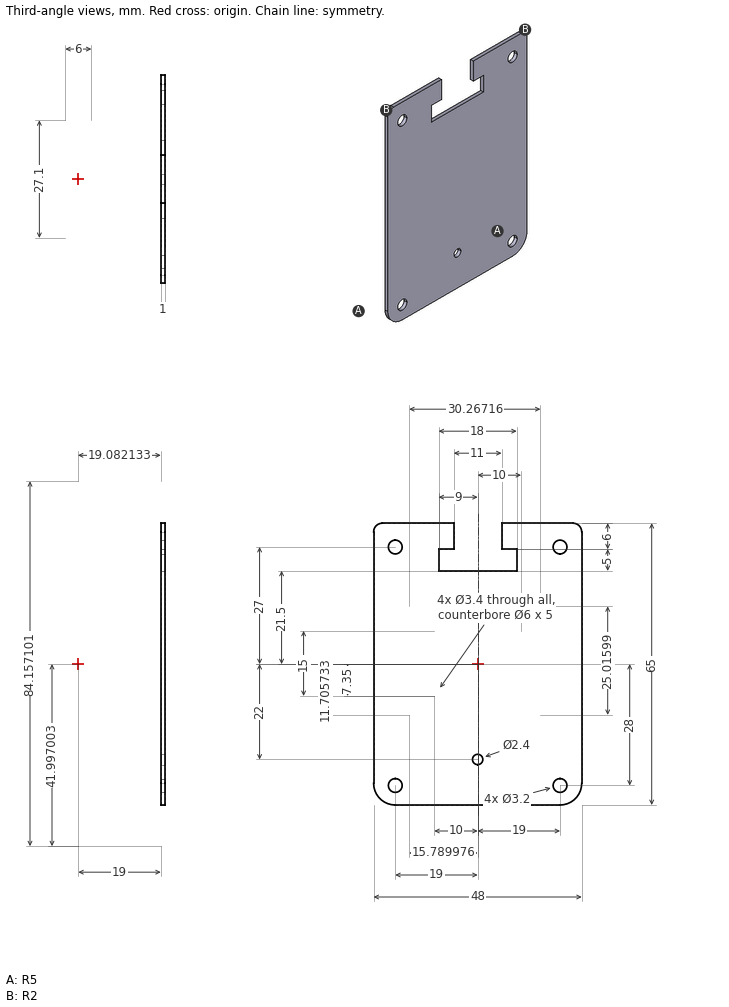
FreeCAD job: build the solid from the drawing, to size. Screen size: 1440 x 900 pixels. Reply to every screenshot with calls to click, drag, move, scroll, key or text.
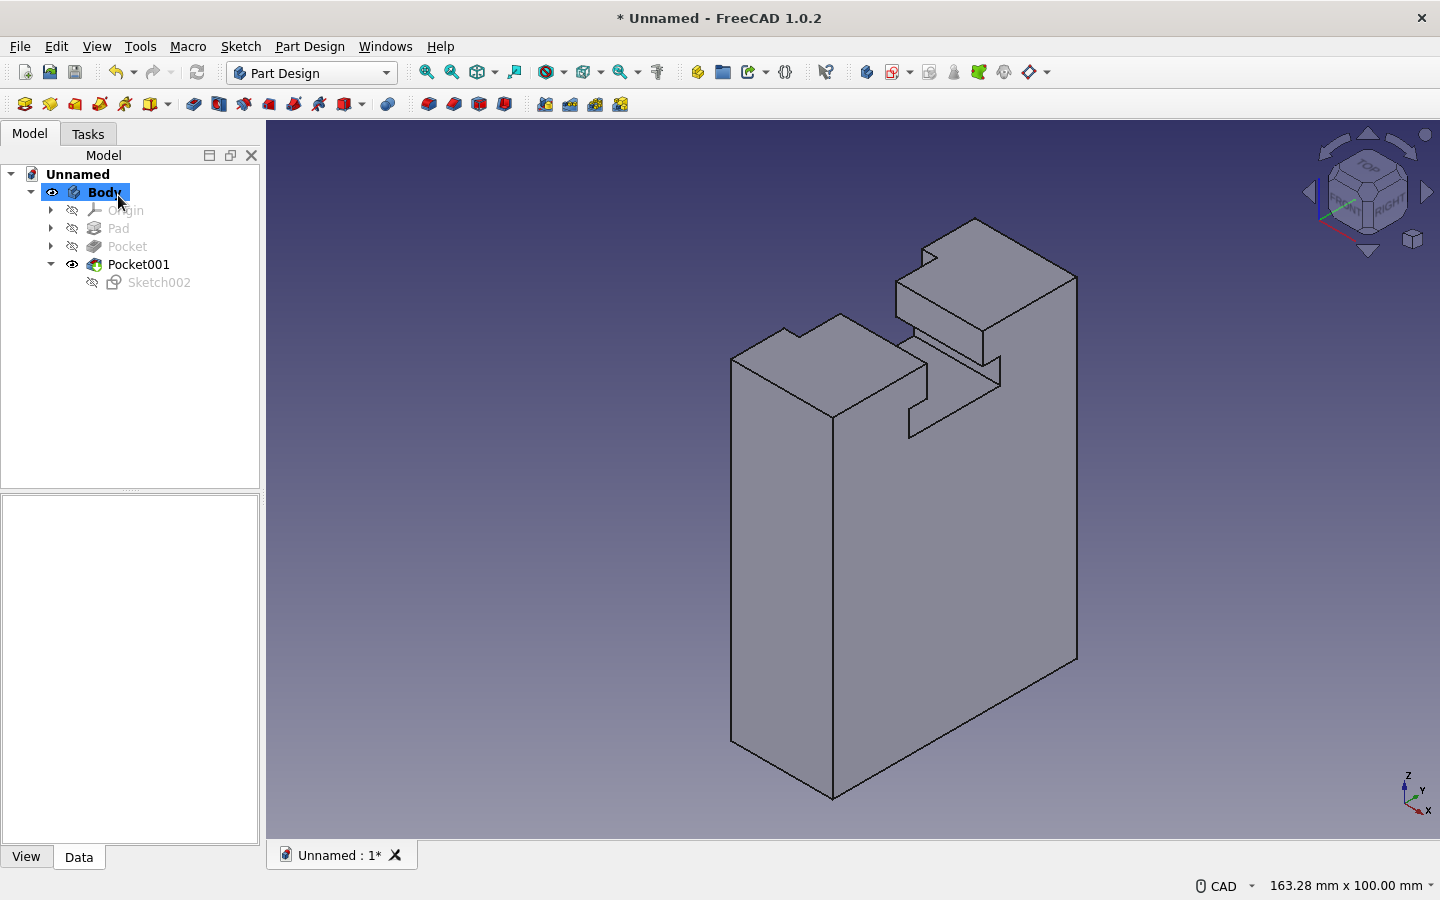
click(955, 592)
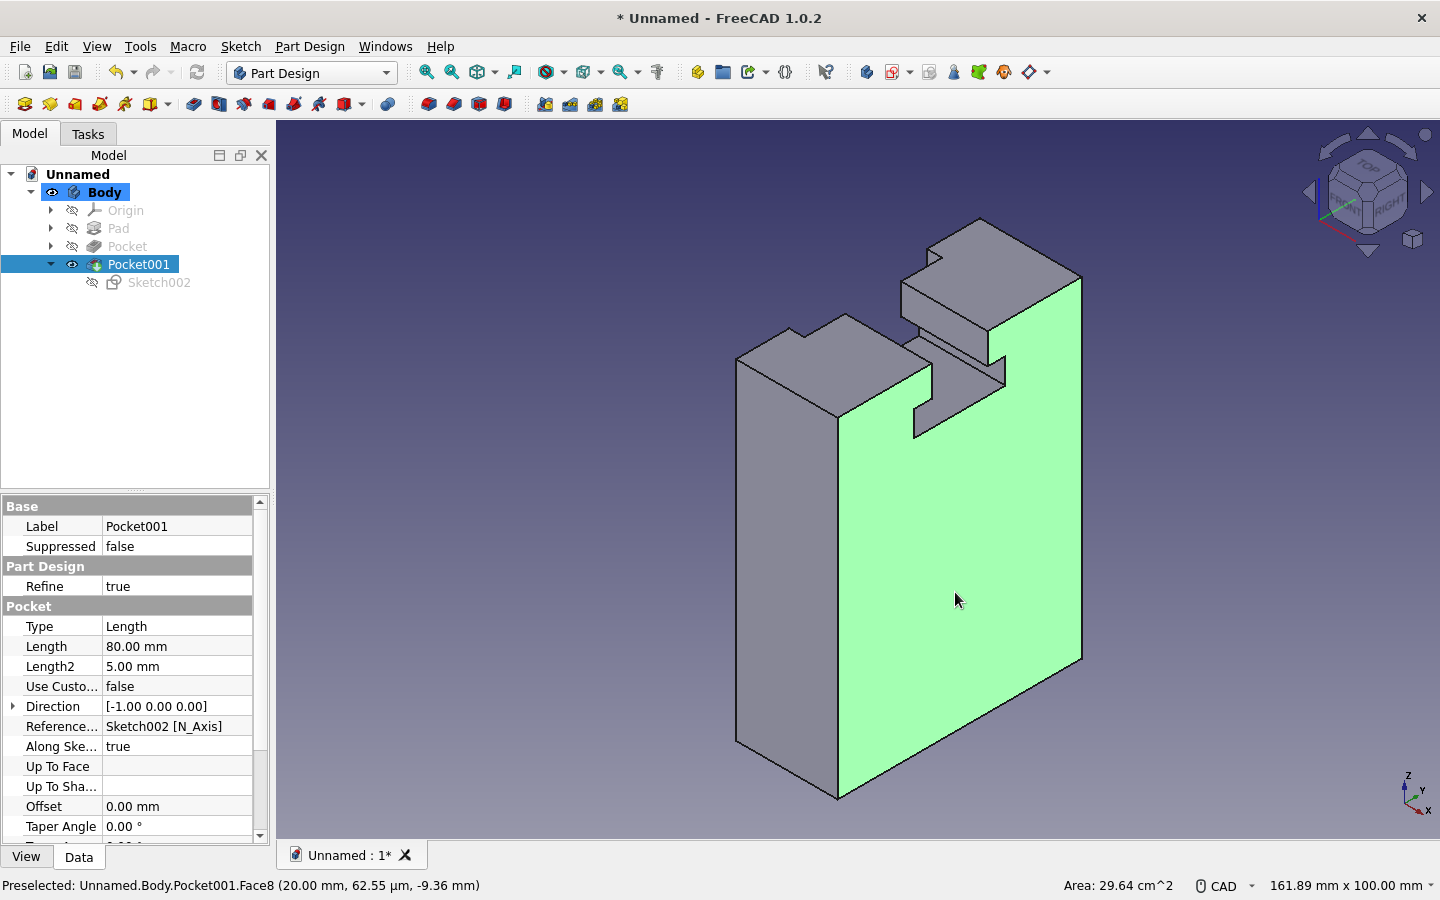
click(892, 72)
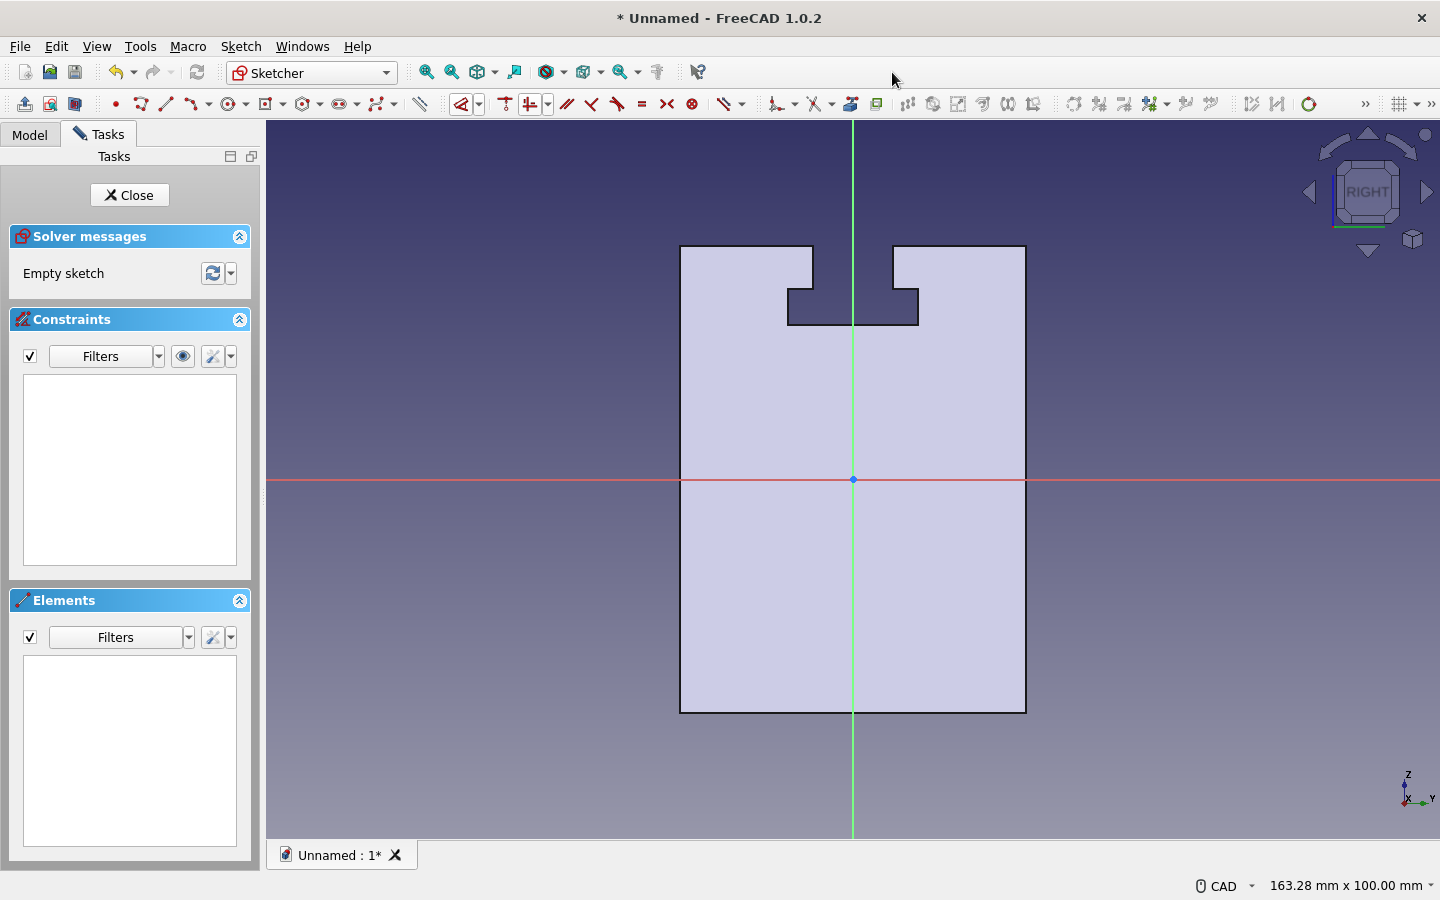
scroll(857, 646, up, 15)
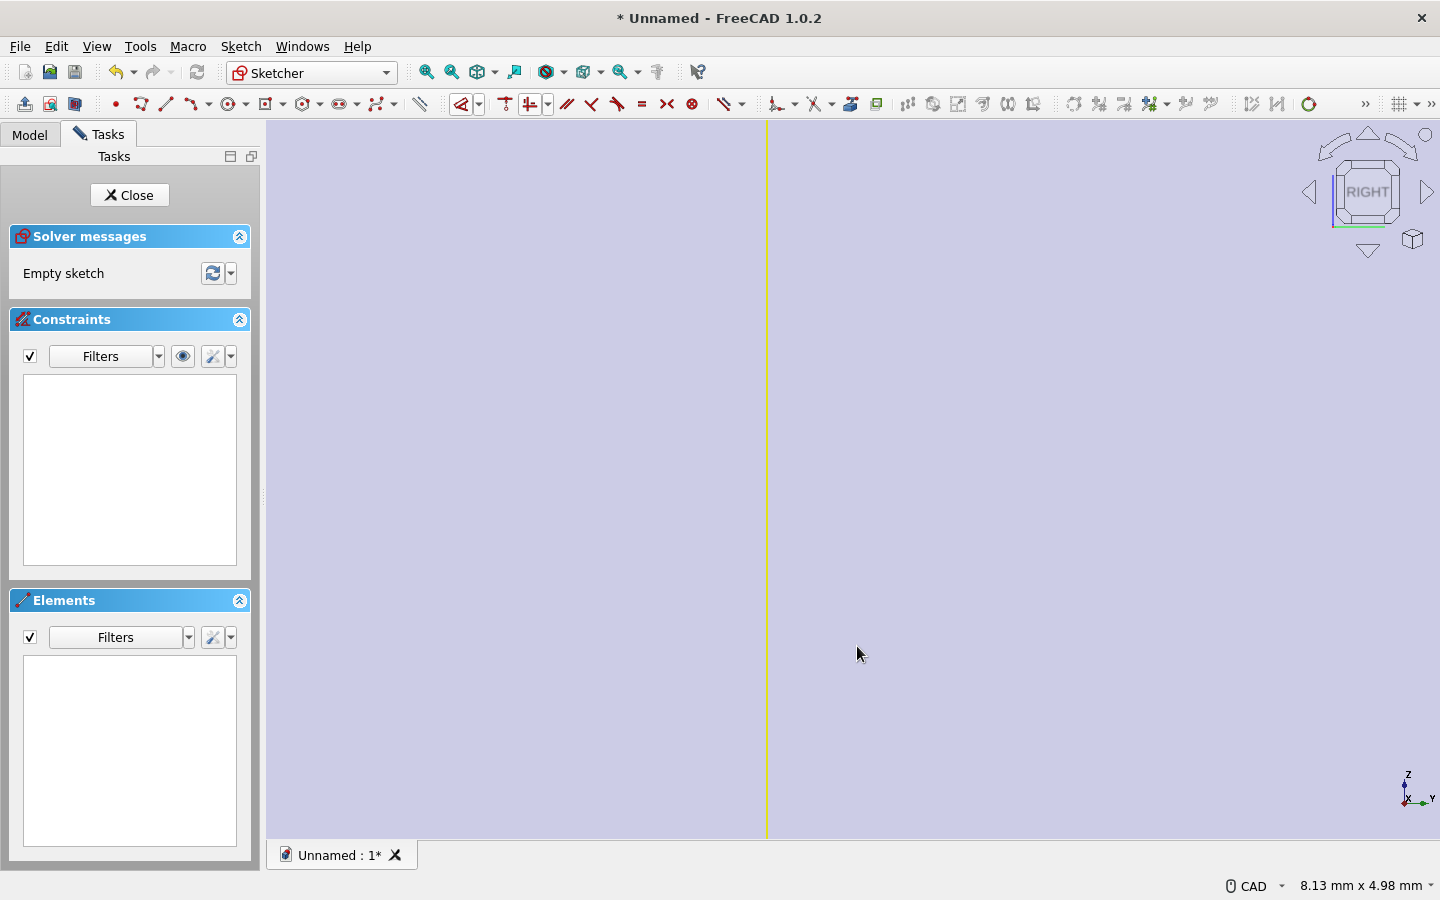
scroll(732, 435, up, 2)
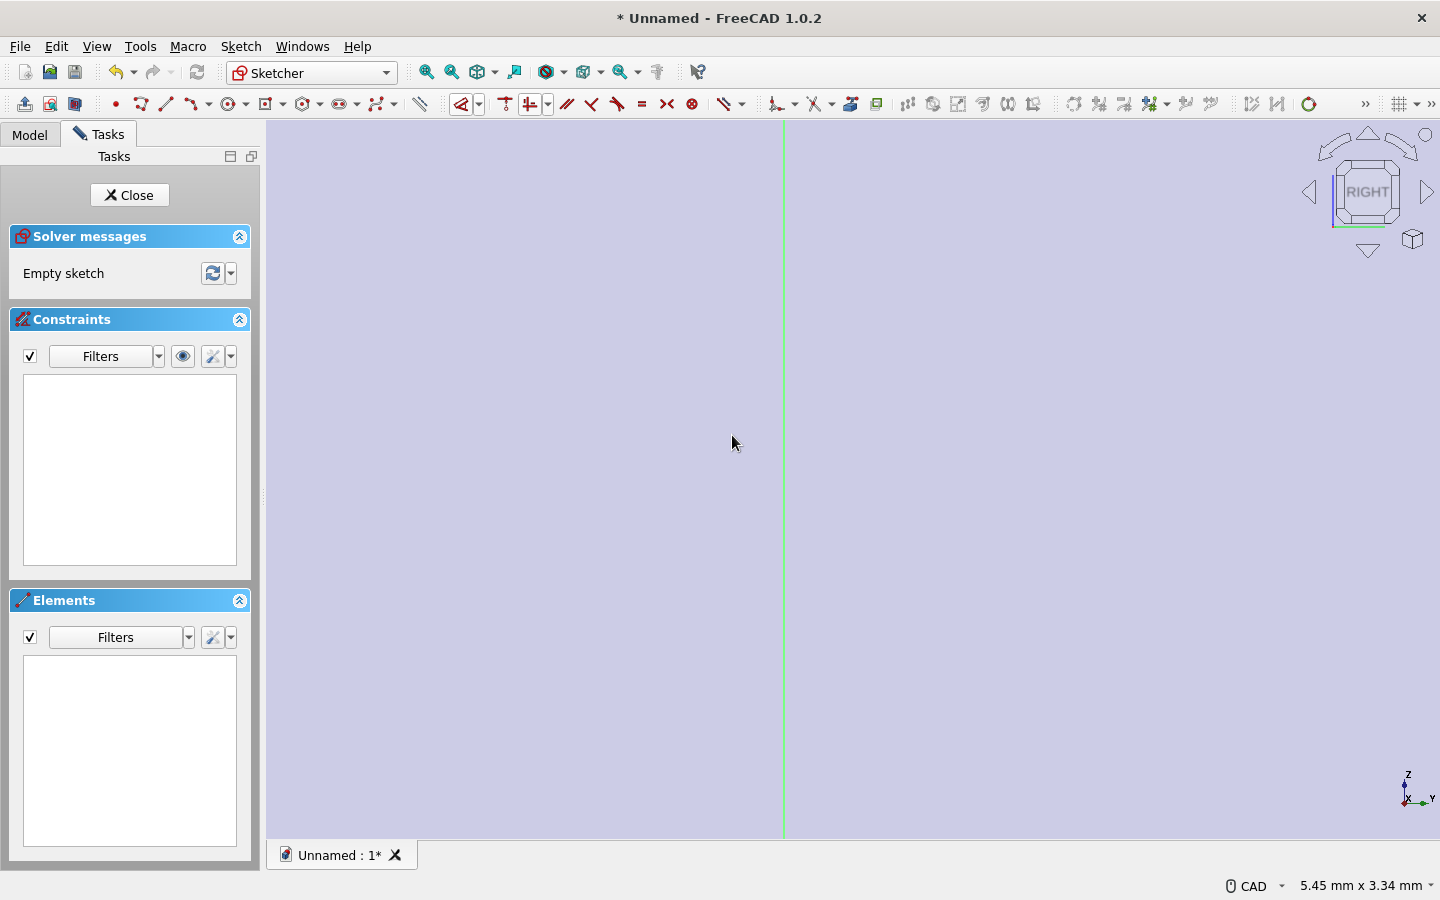
key(g)
key(c)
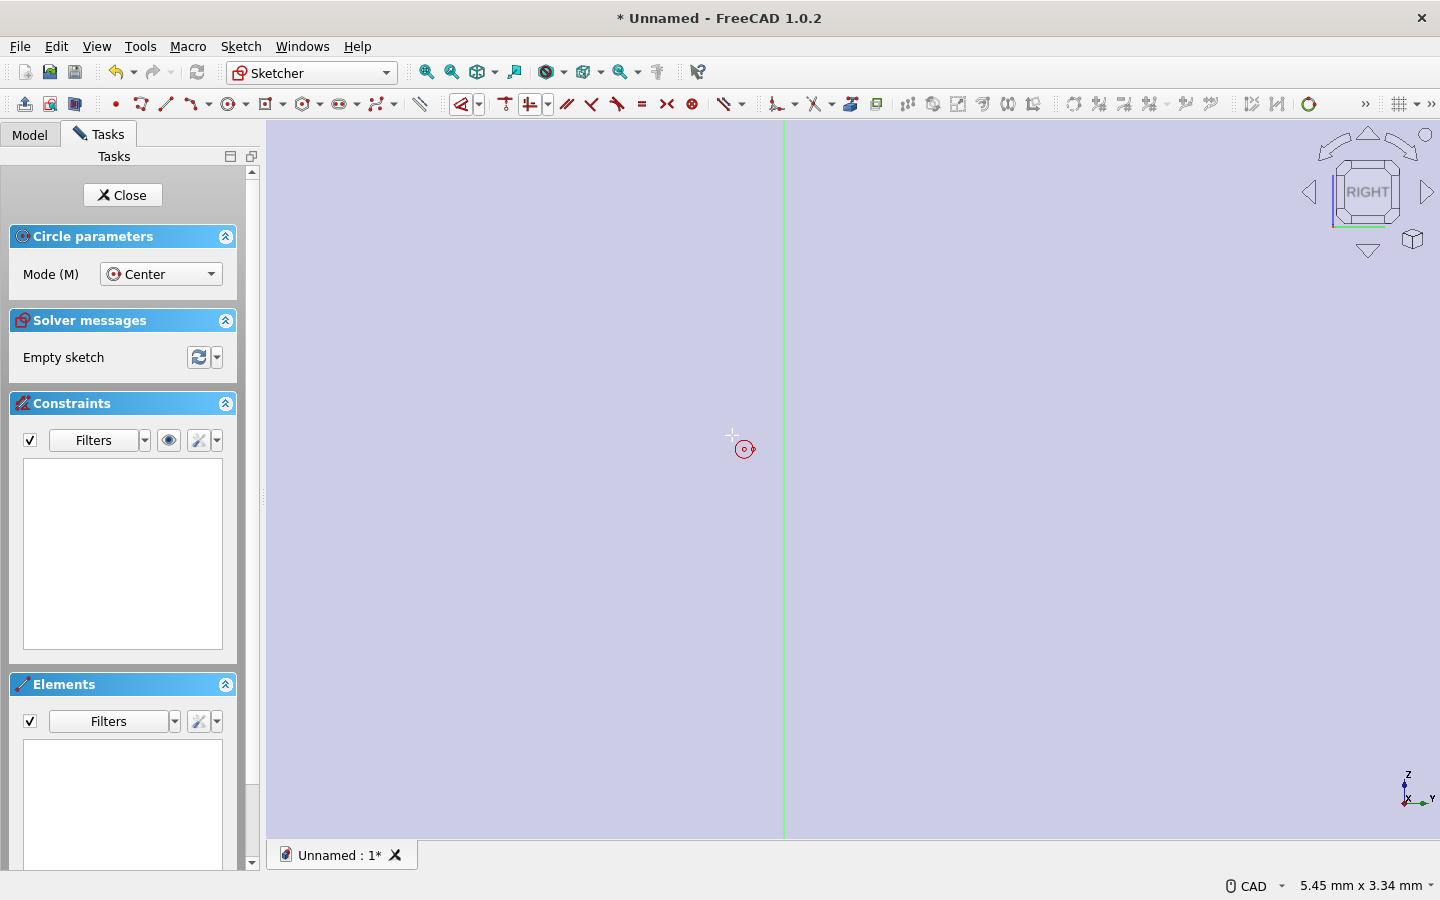
click(784, 479)
move(967, 297)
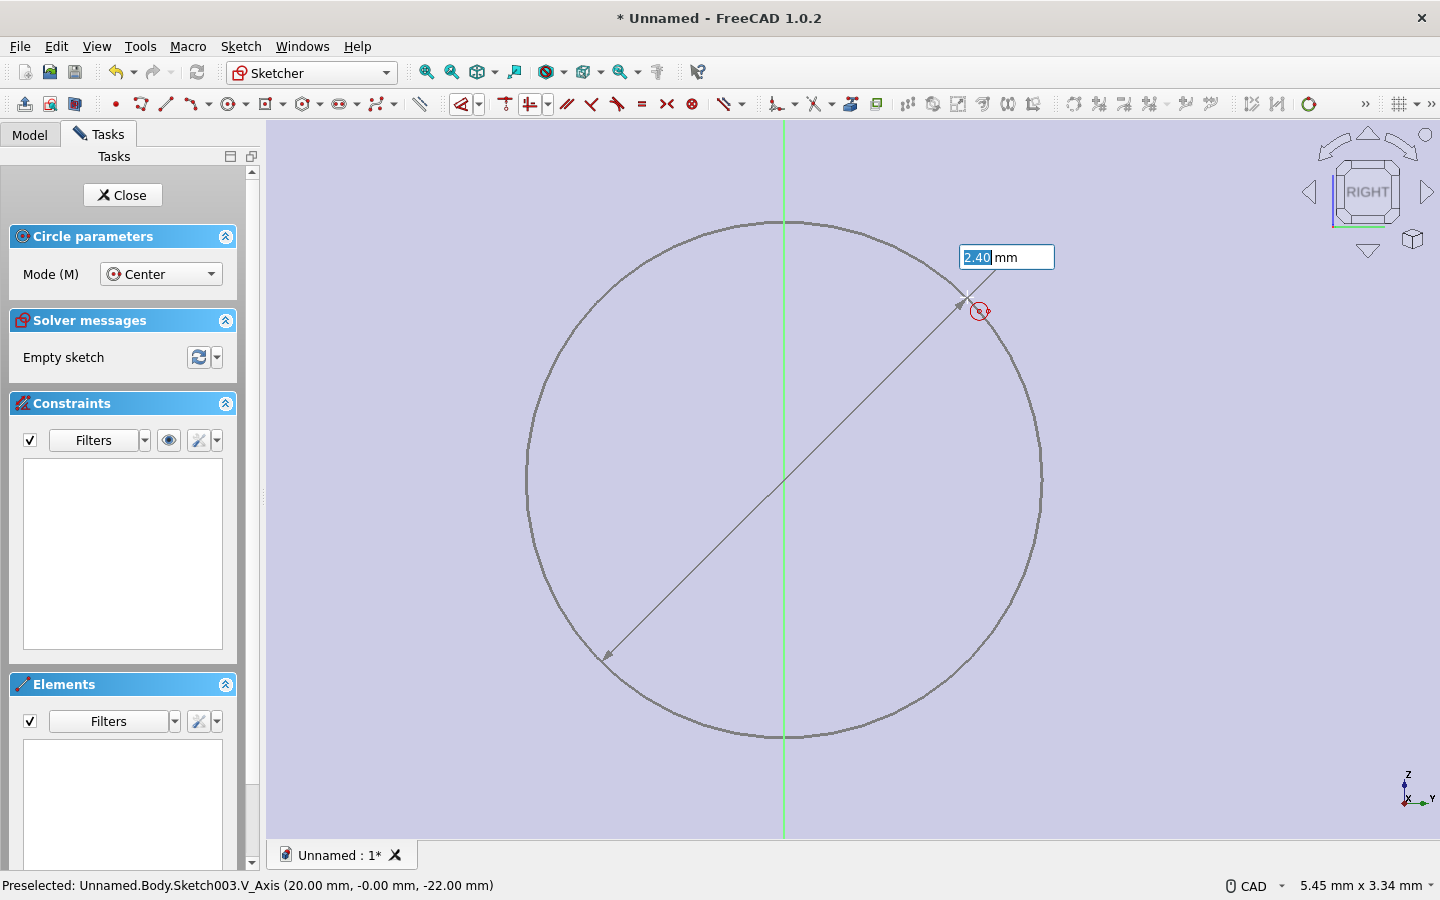
text(2.4)
key(Return)
key(Escape)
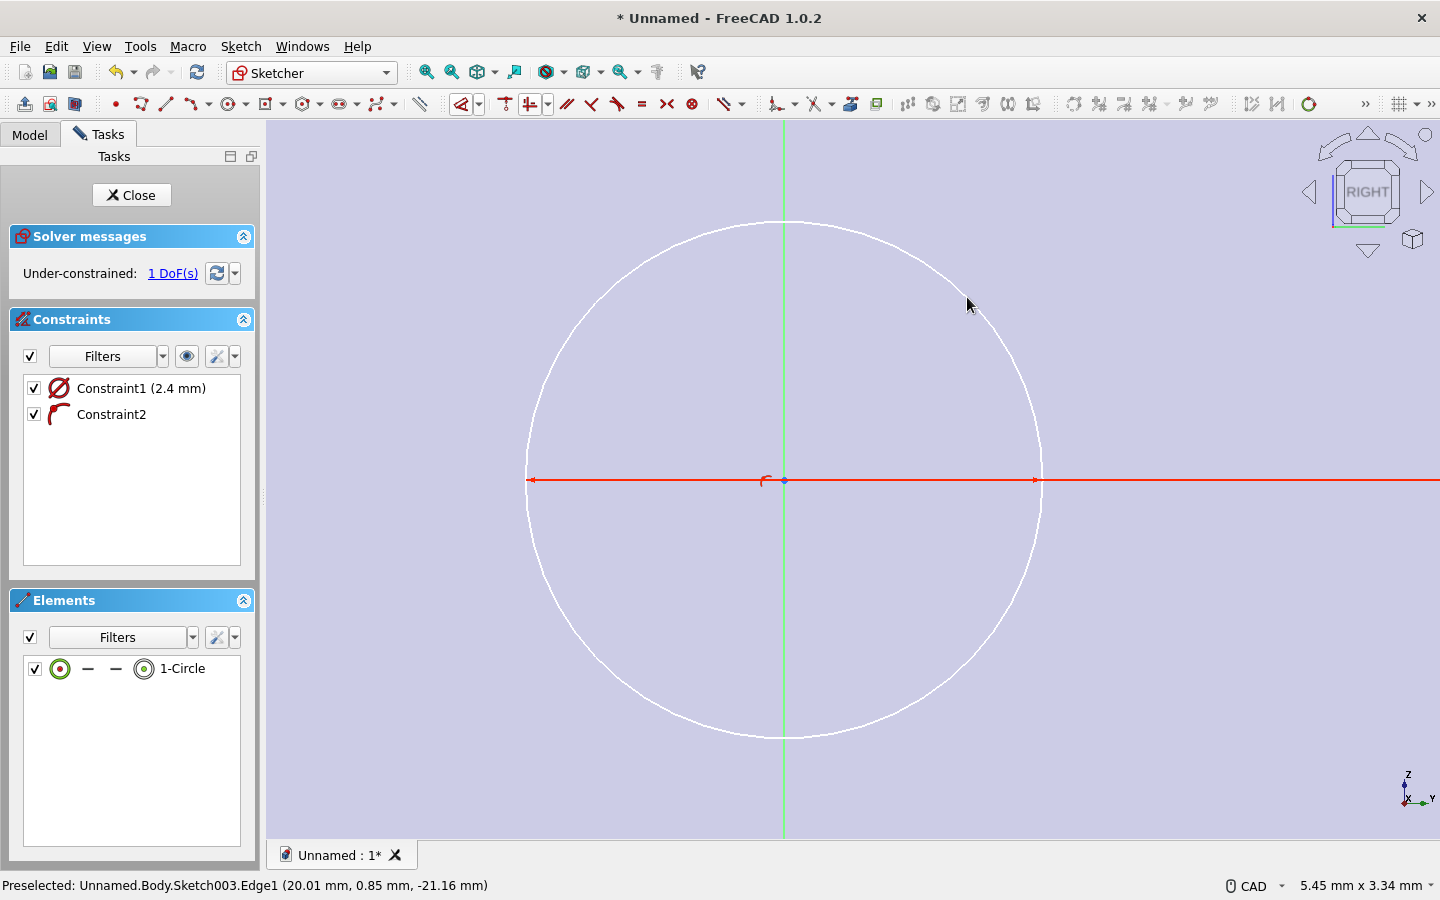
click(784, 480)